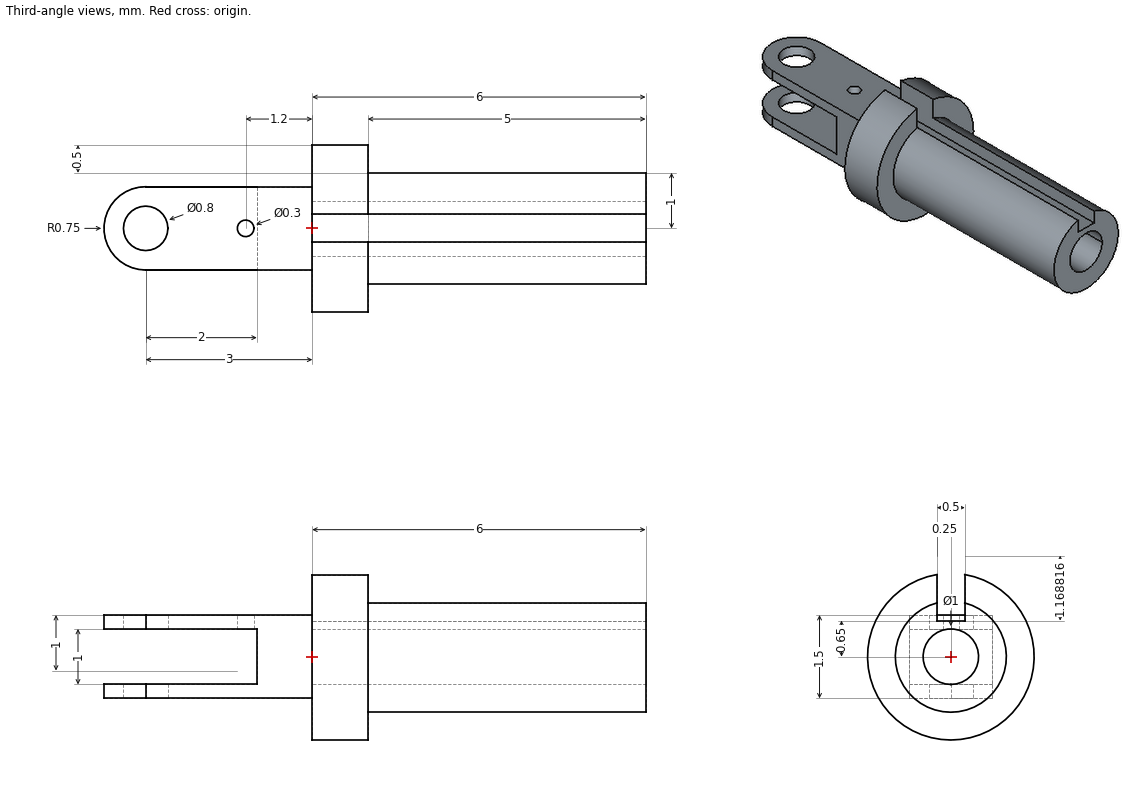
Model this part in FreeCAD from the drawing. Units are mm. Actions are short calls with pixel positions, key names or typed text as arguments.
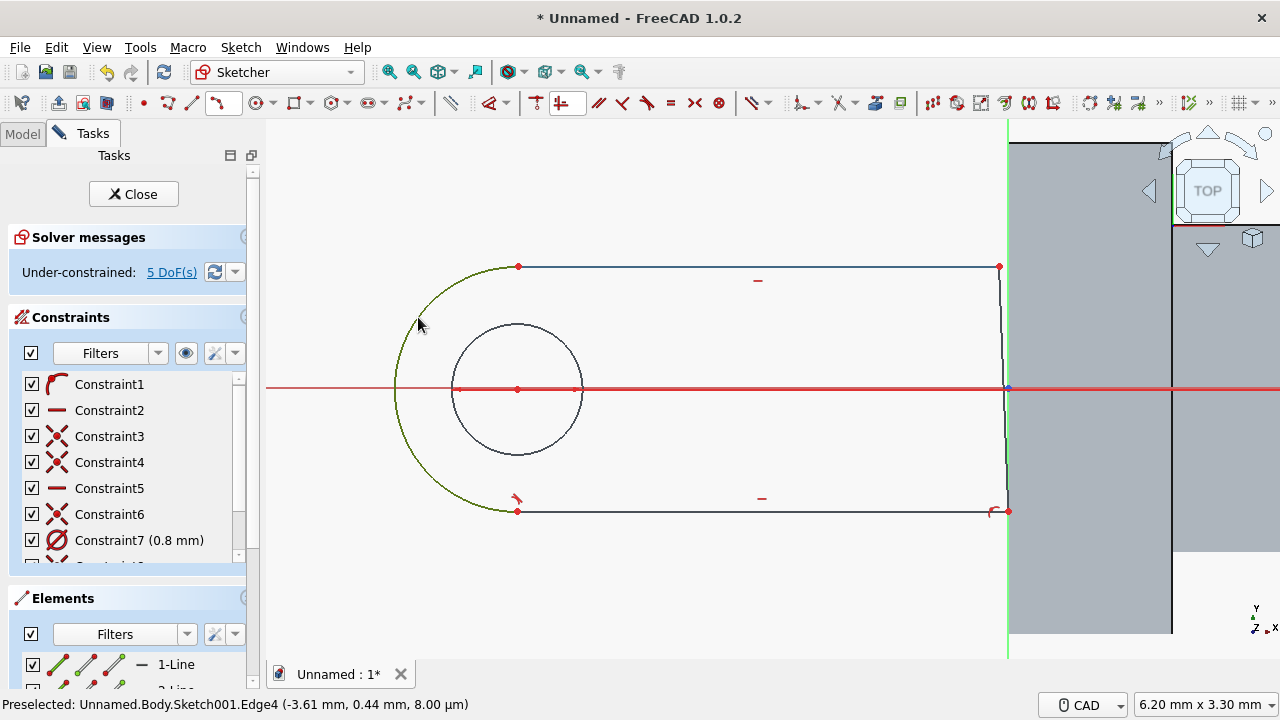
click(648, 104)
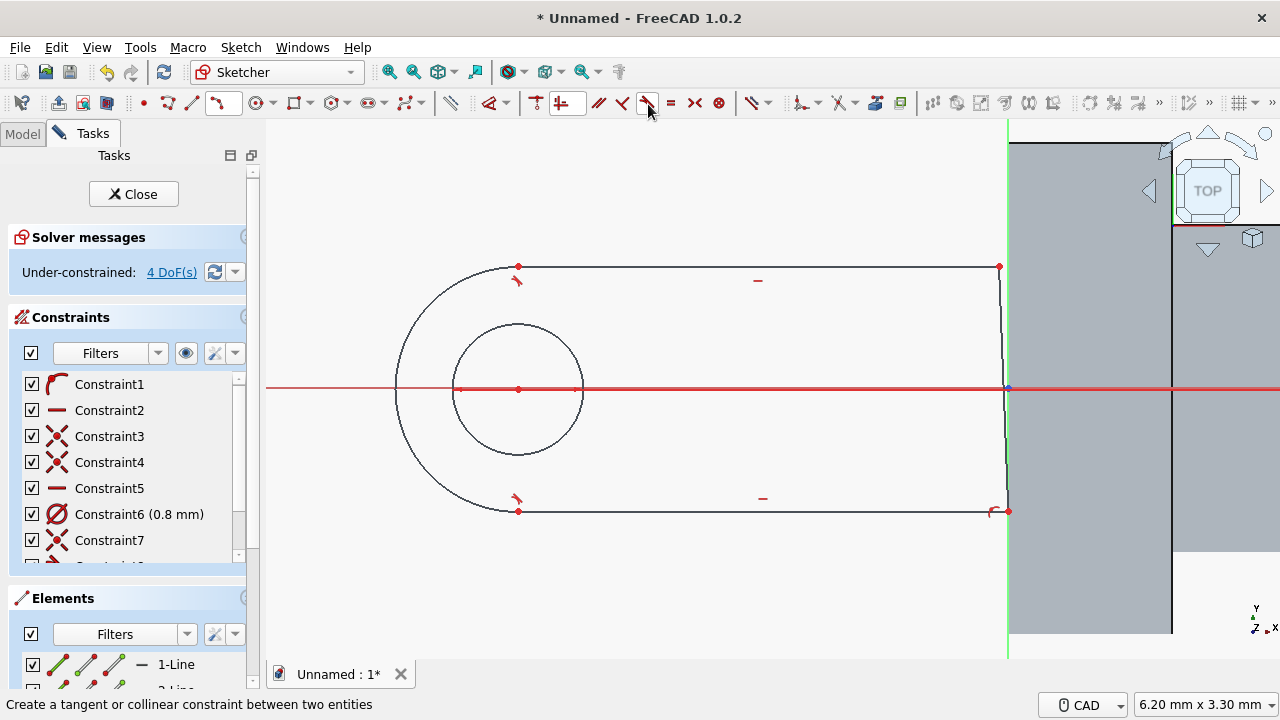
click(1006, 438)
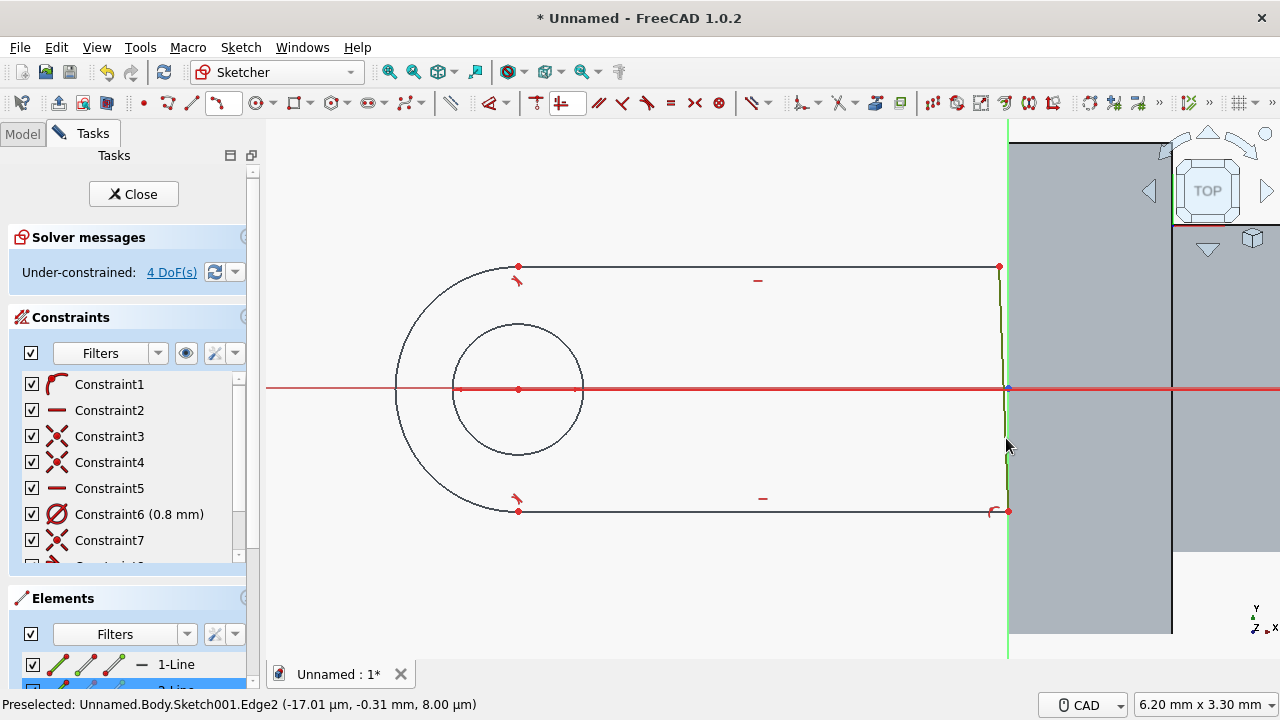
key(v)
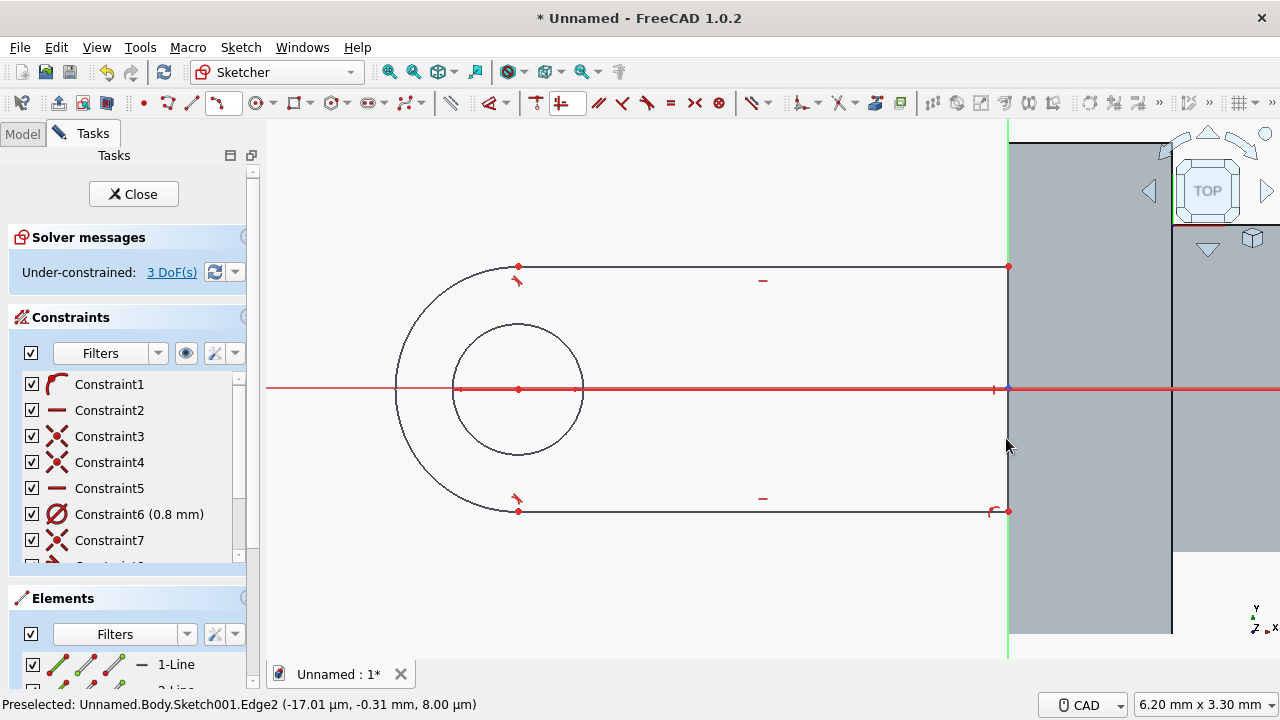
click(518, 389)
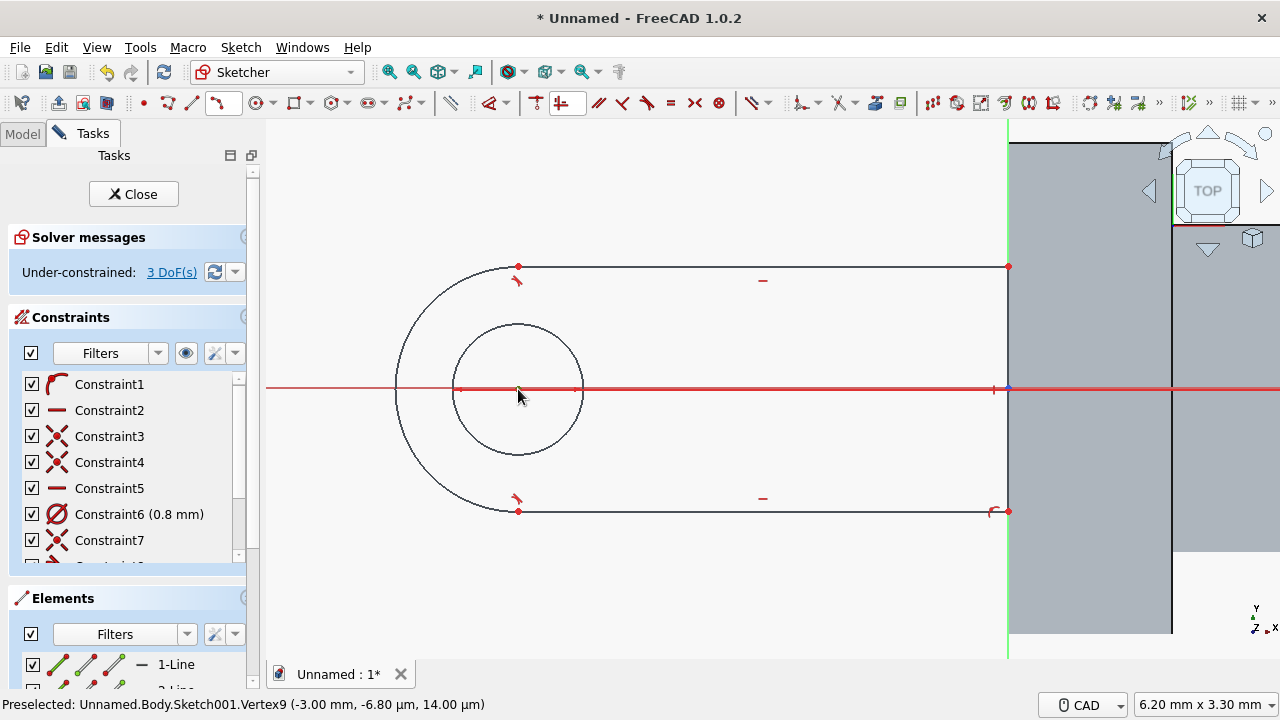
click(353, 388)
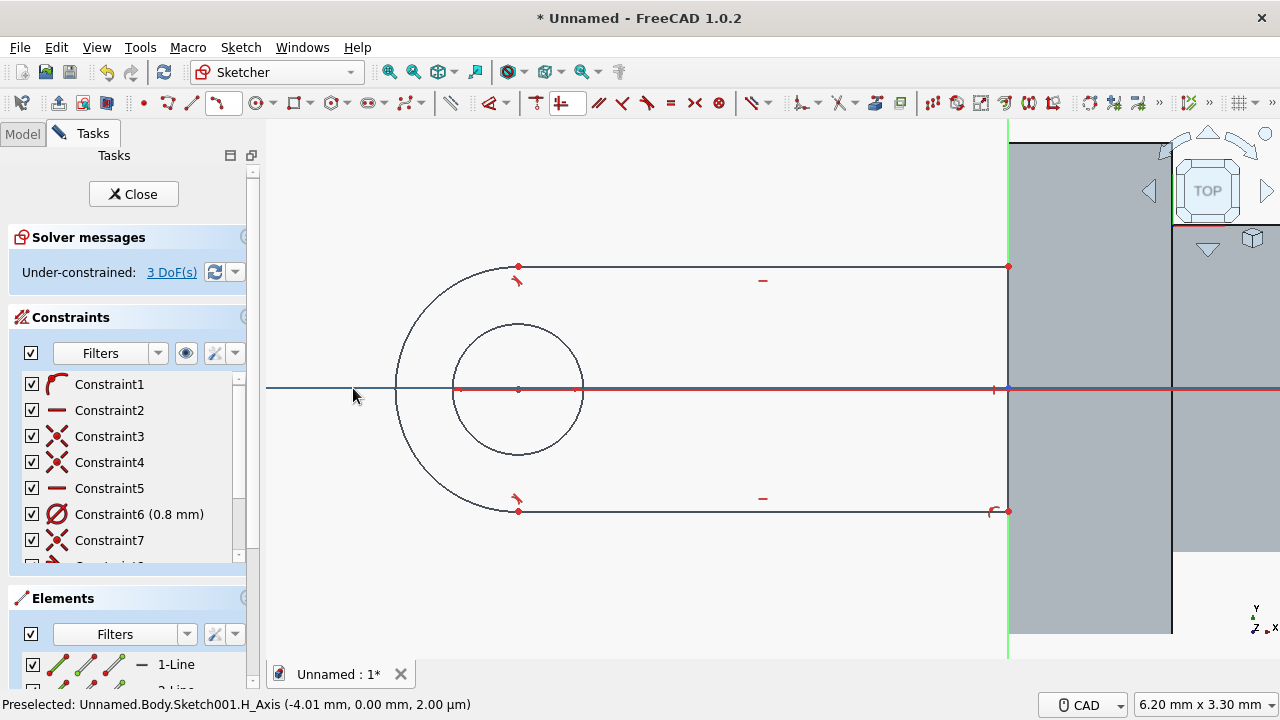
click(536, 104)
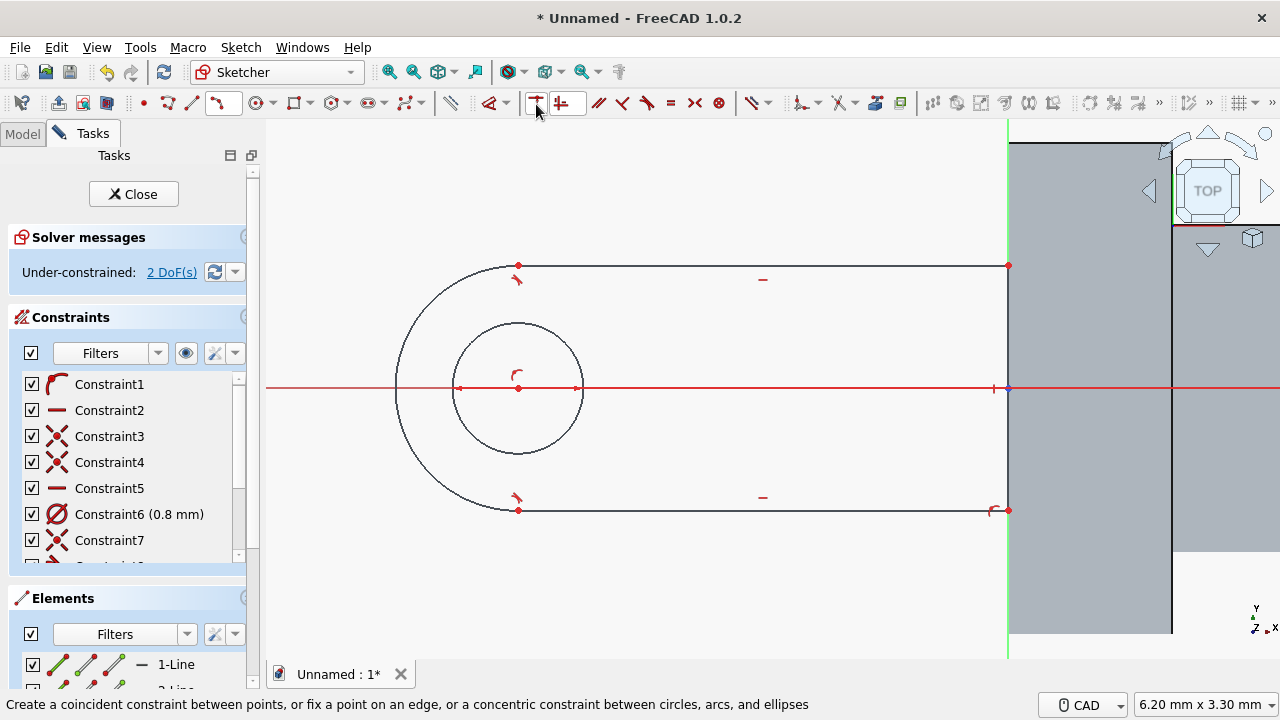
click(490, 104)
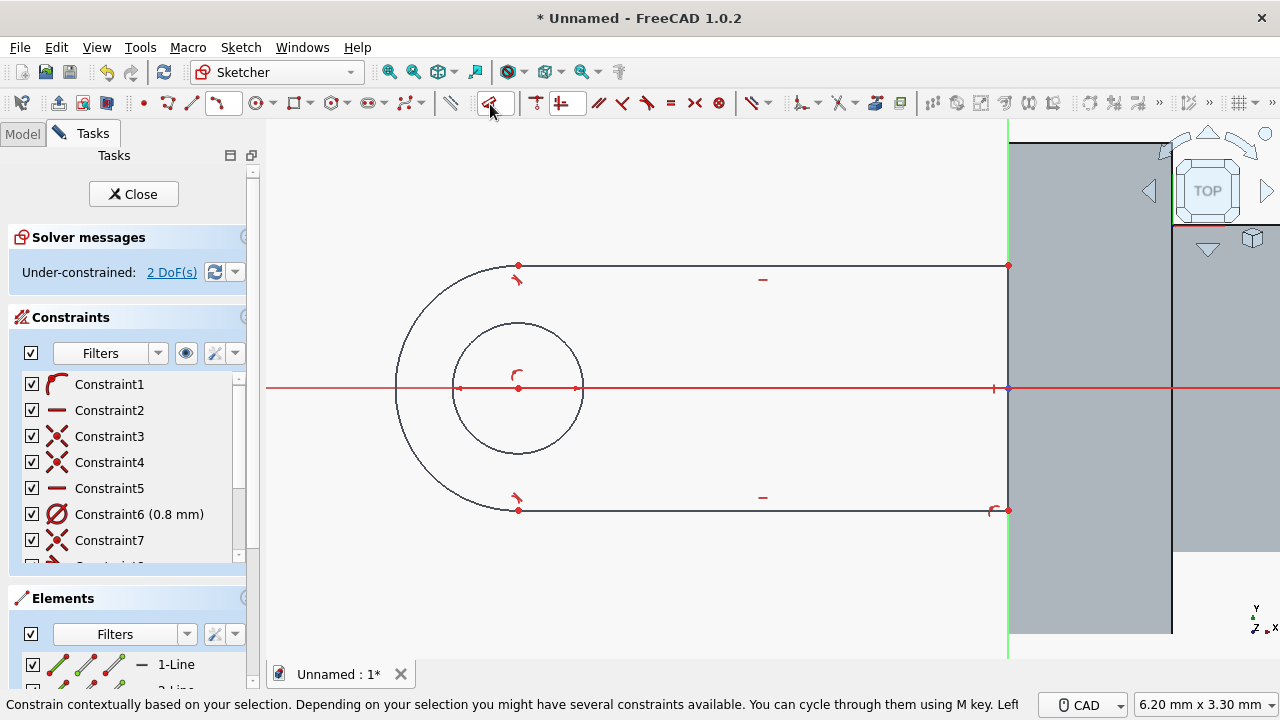
click(419, 316)
click(393, 297)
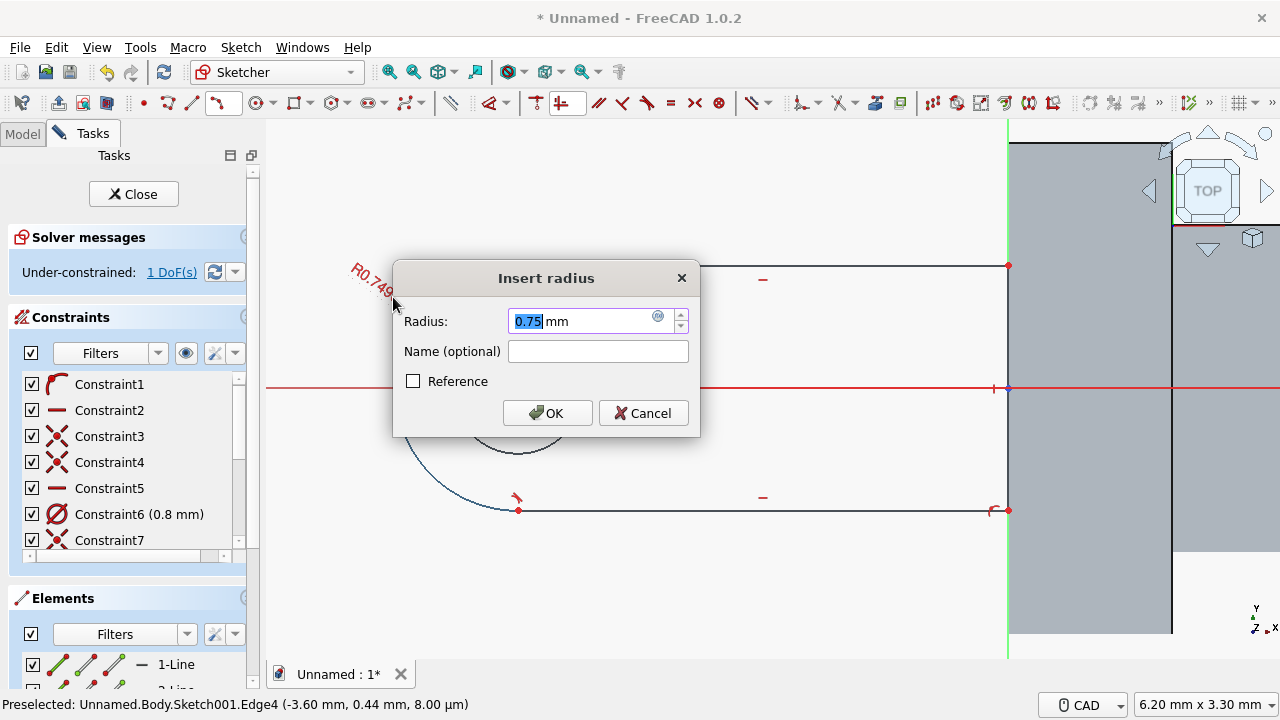
text(0.75)
key(Return)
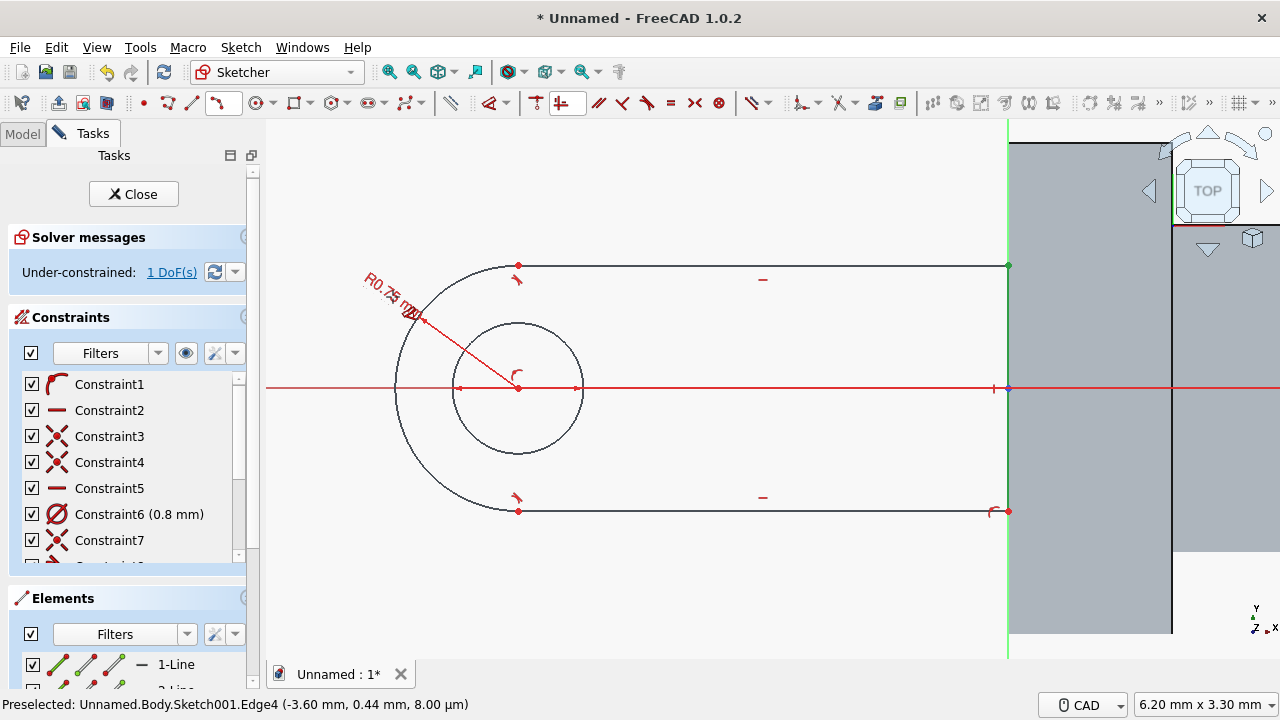
click(665, 511)
click(763, 545)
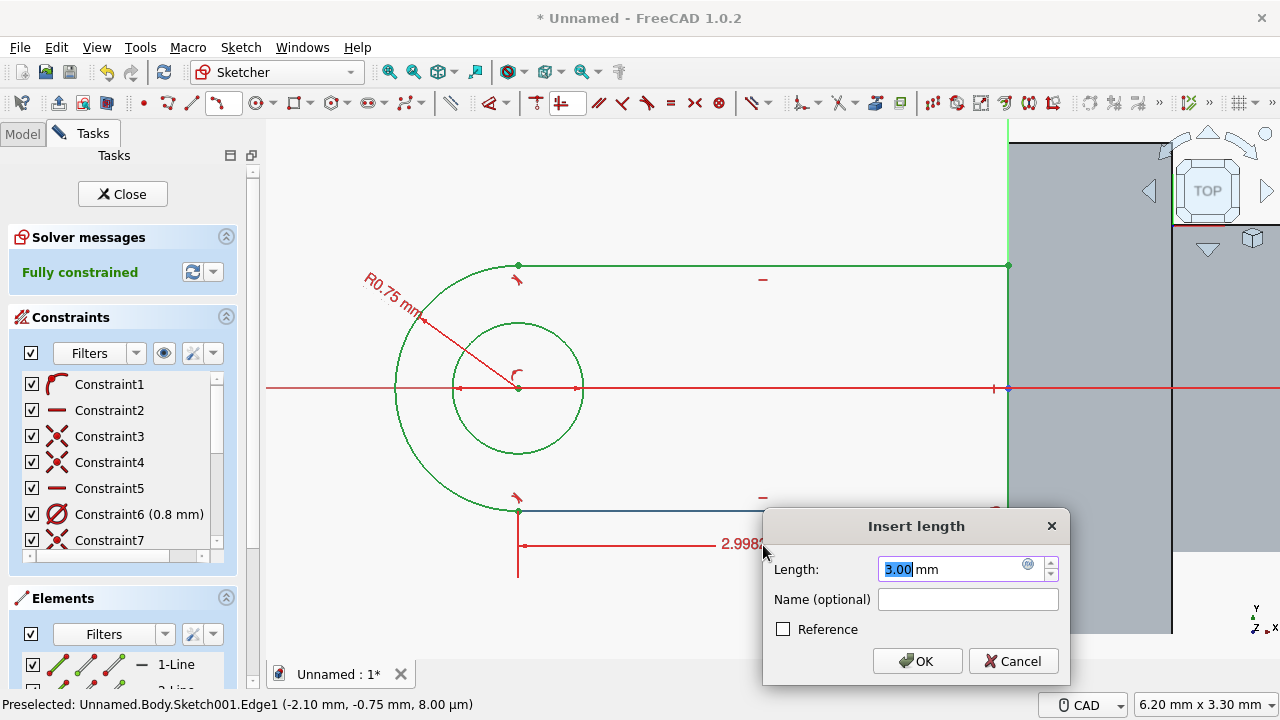
text(3)
key(Return)
key(Escape)